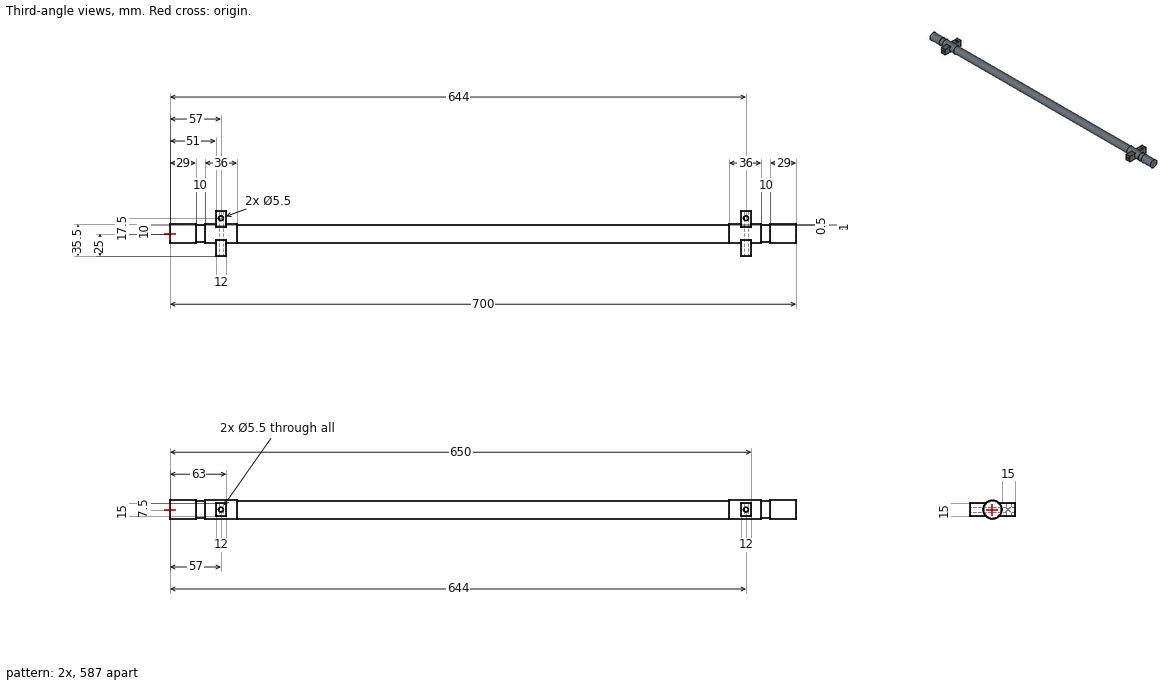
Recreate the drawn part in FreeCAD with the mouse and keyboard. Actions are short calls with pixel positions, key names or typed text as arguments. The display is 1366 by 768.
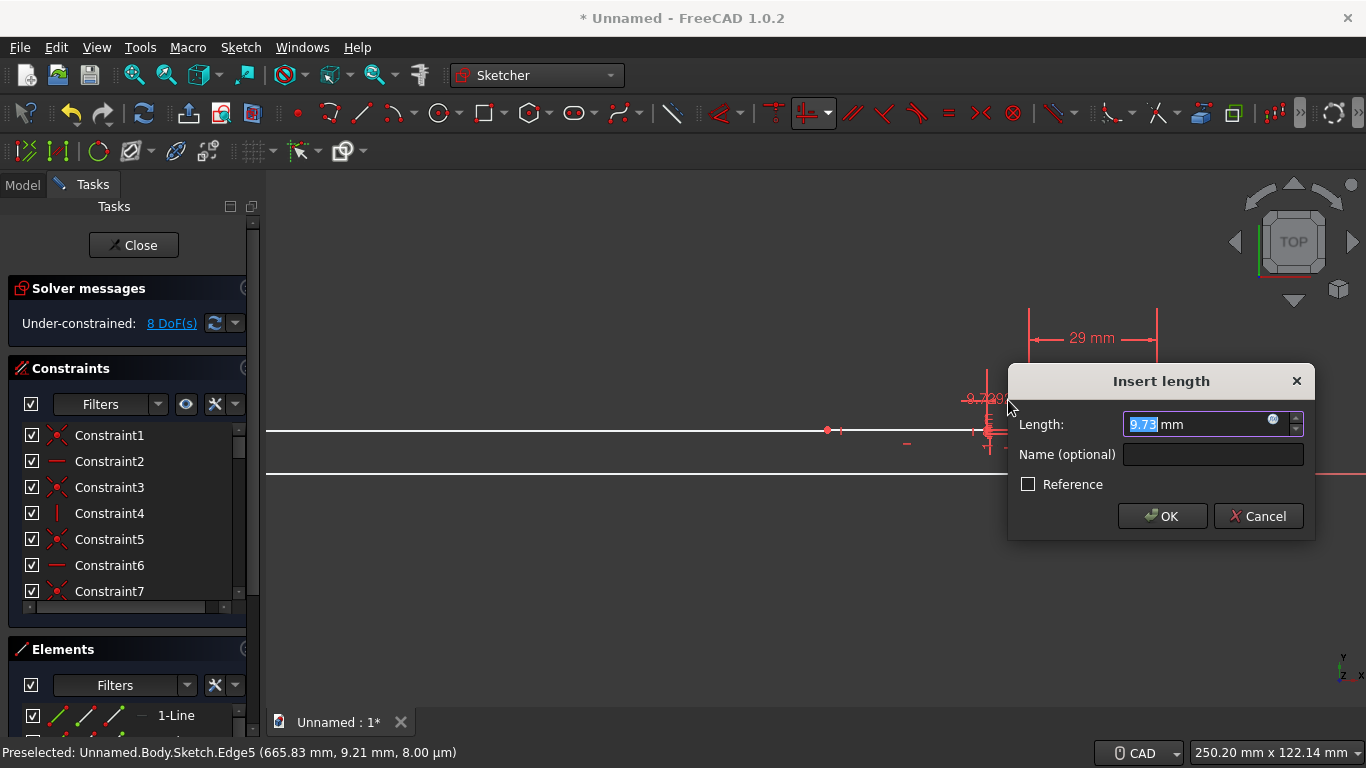
text(10)
key(Return)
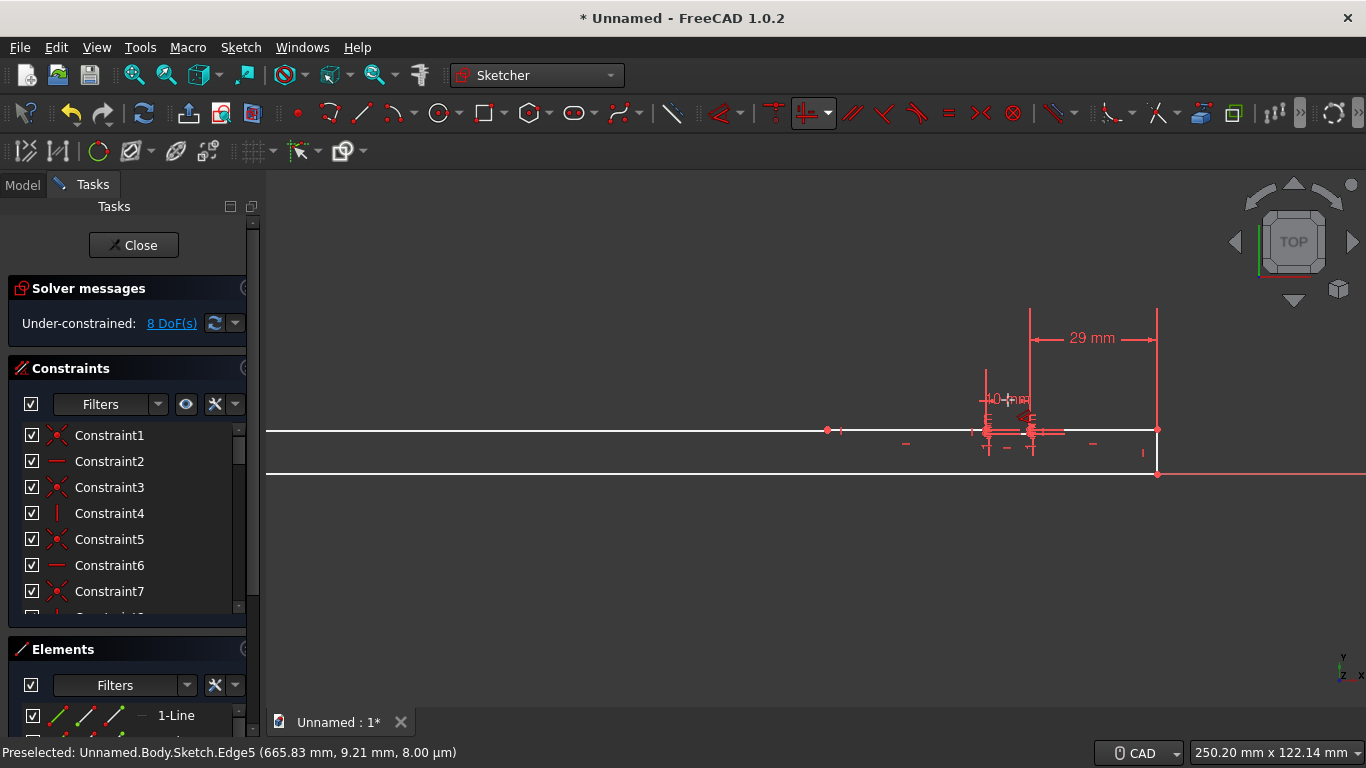
scroll(1033, 435, down, 8)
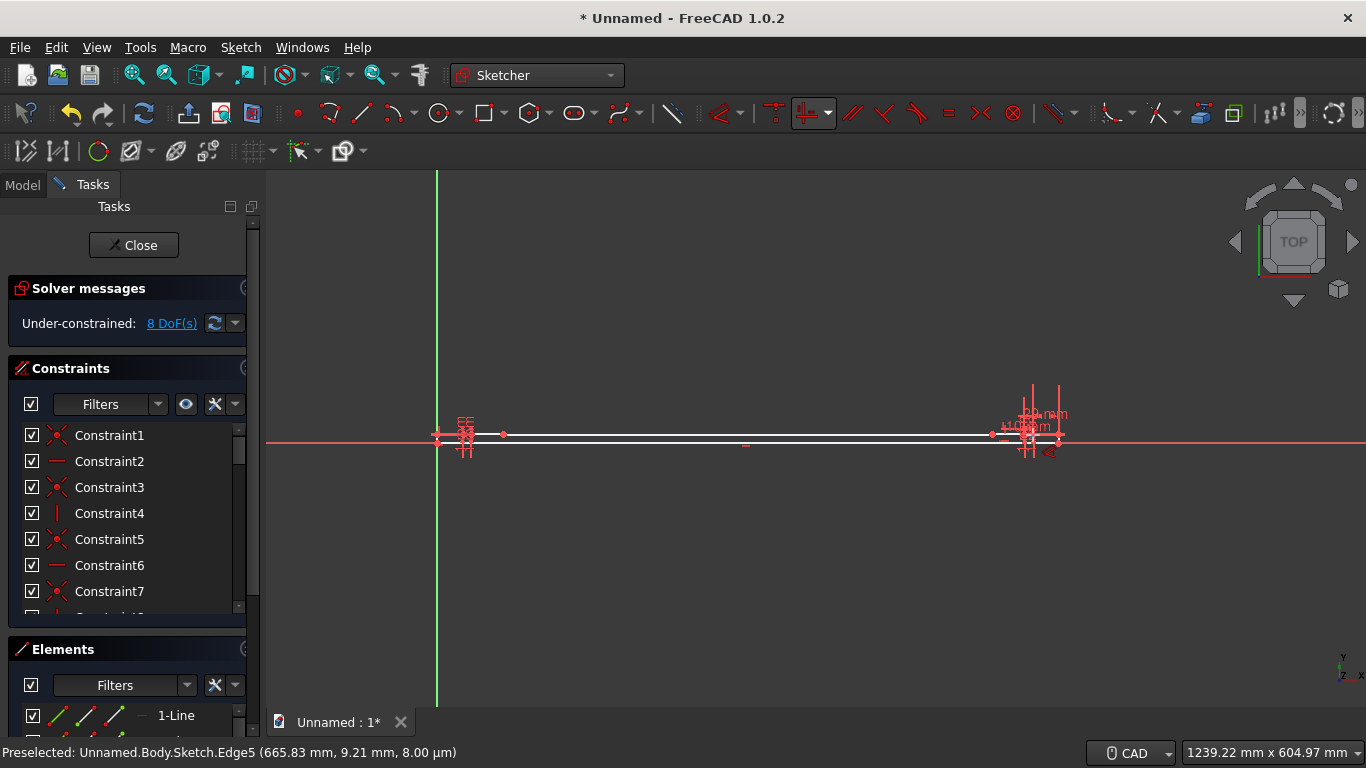
scroll(1014, 434, up, 3)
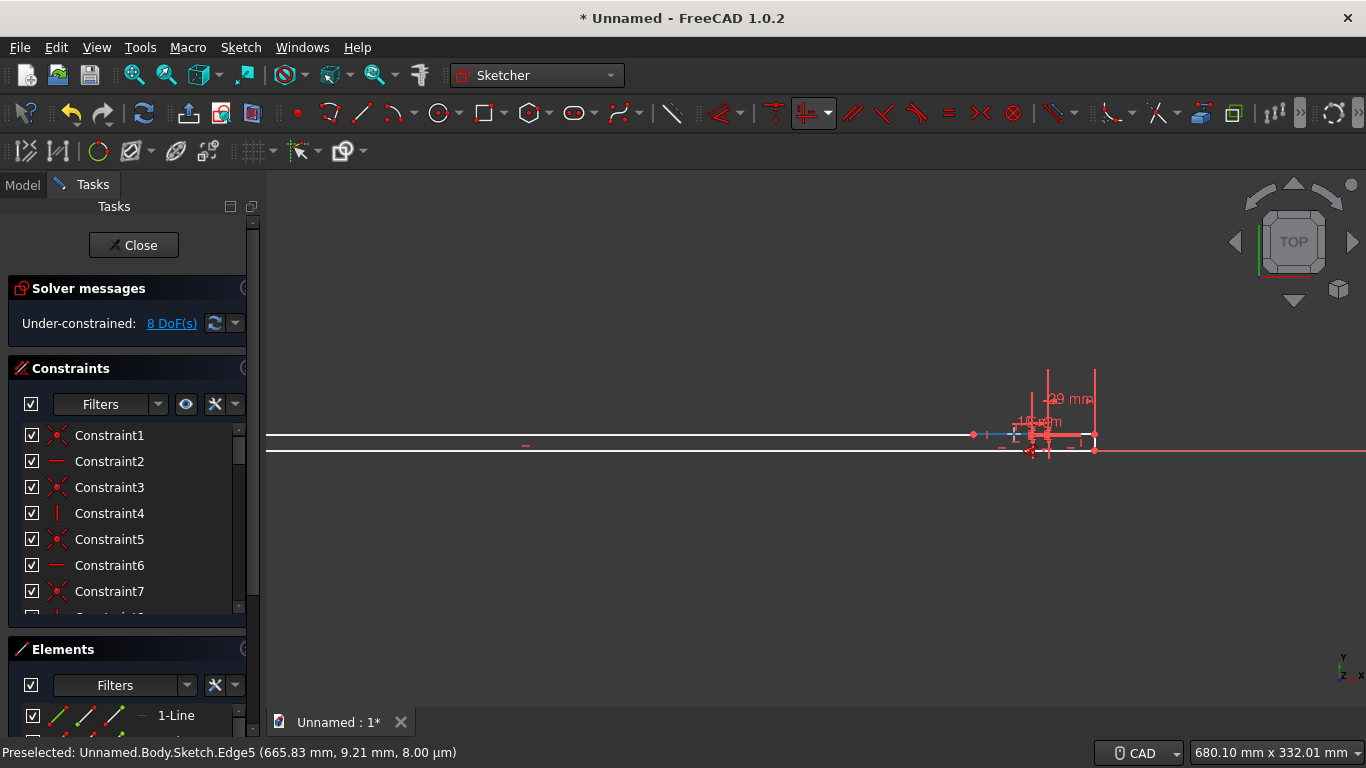
click(1014, 434)
click(989, 400)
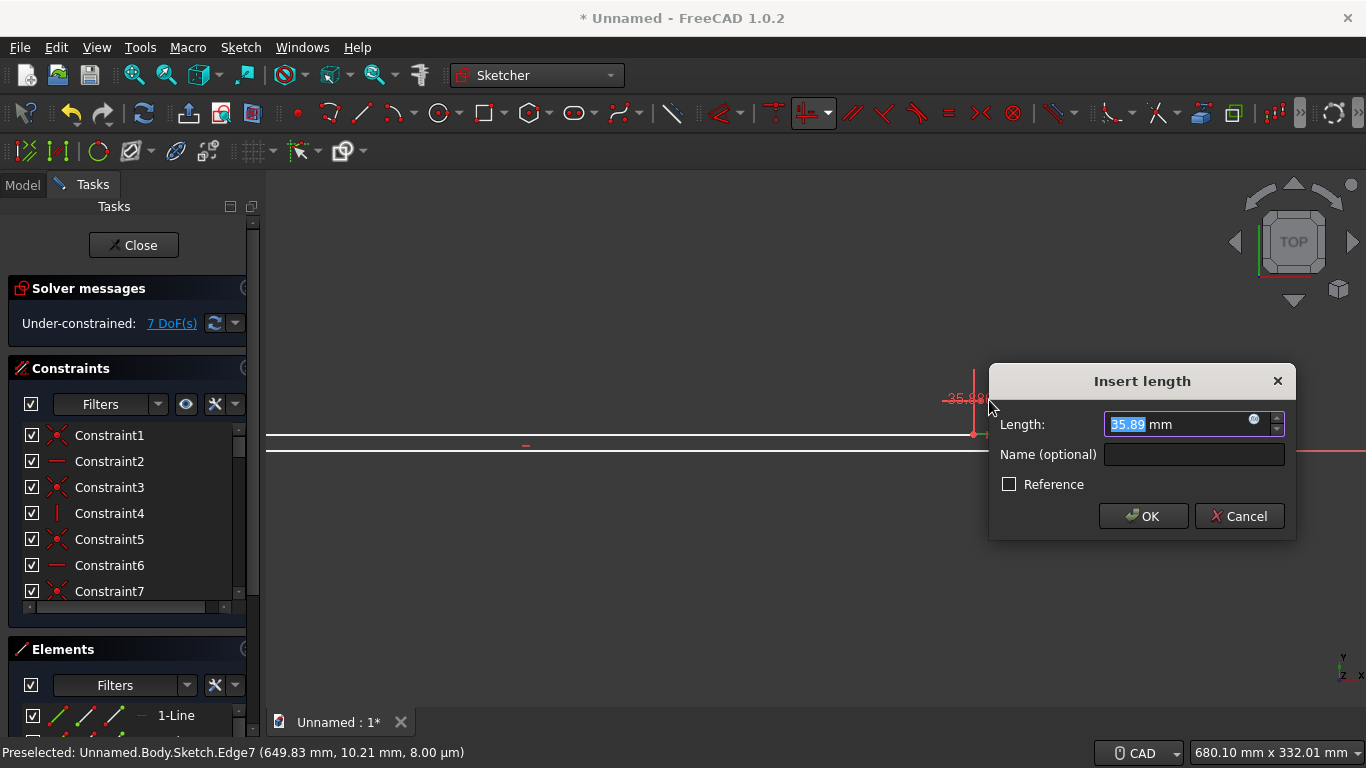
text(36)
key(Return)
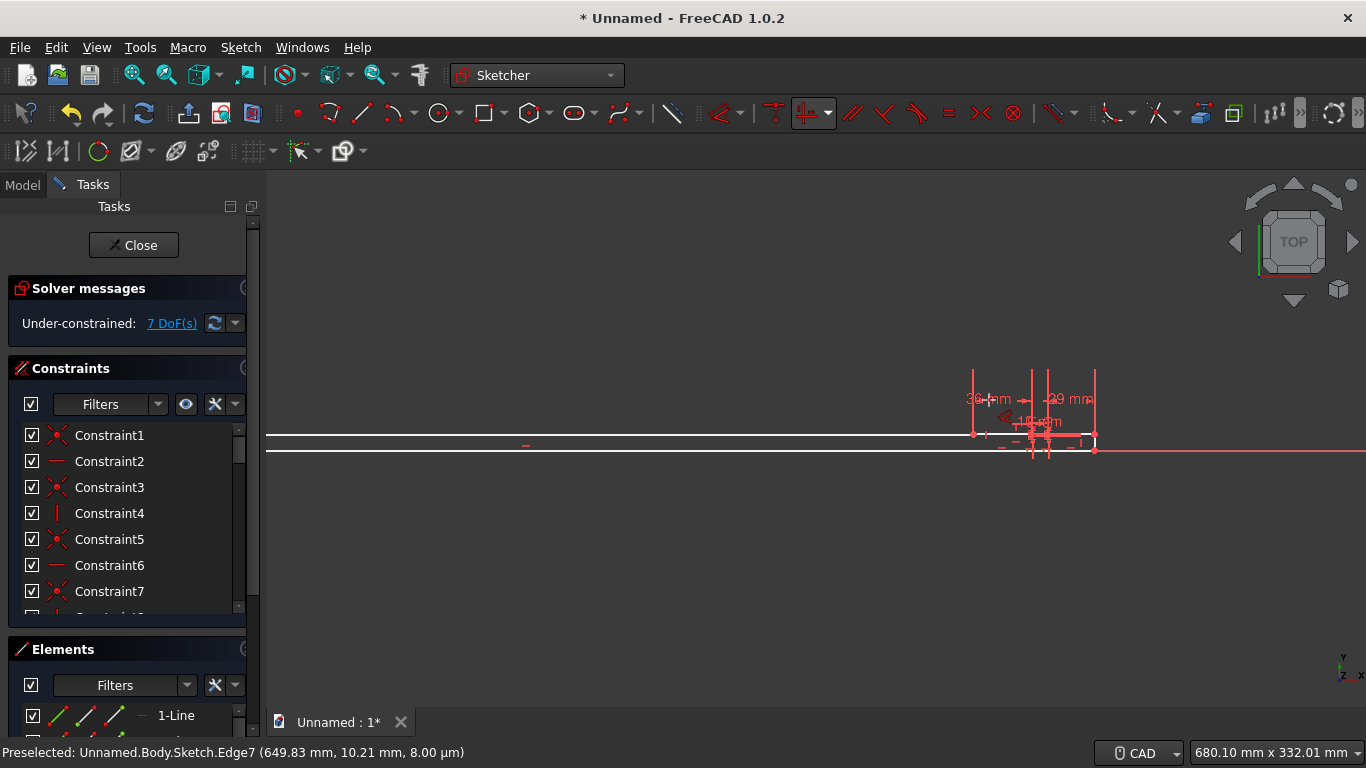
scroll(1013, 434, down, 3)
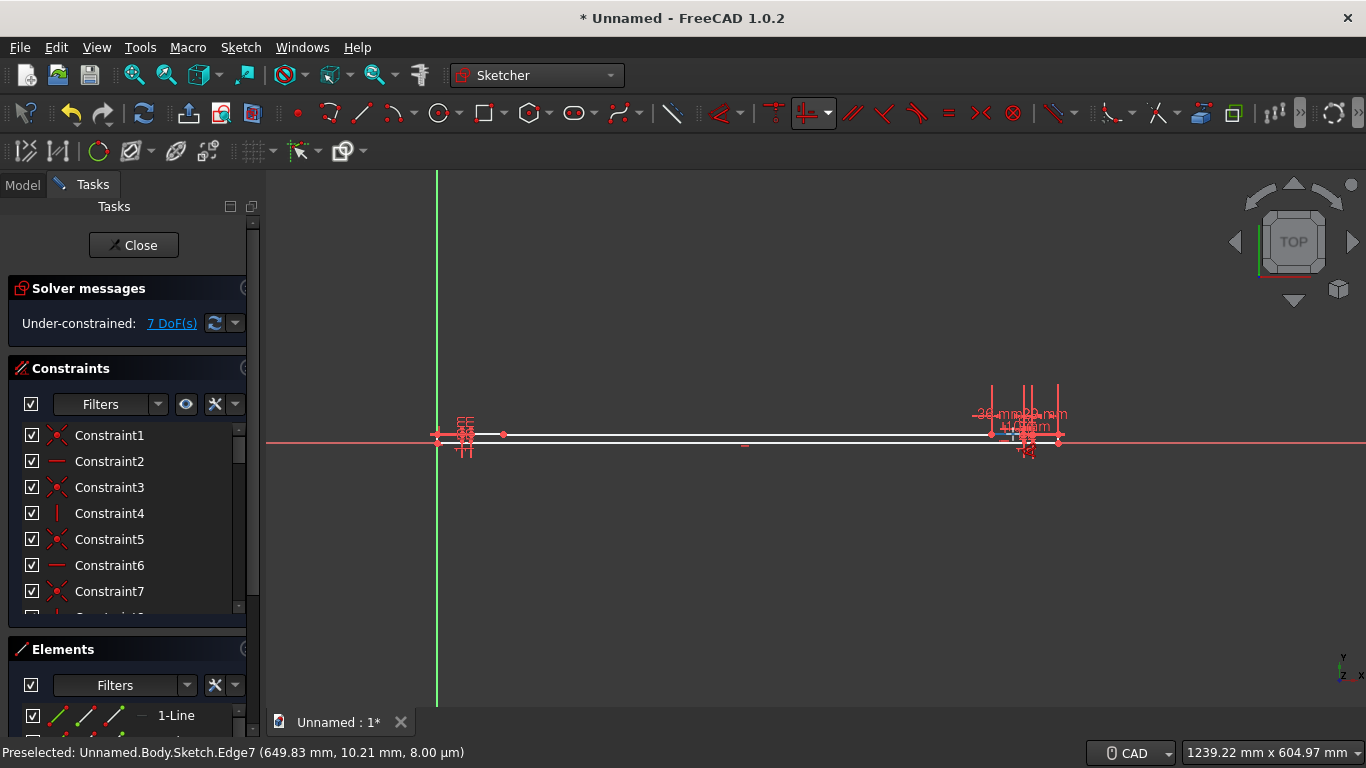
scroll(494, 434, up, 2)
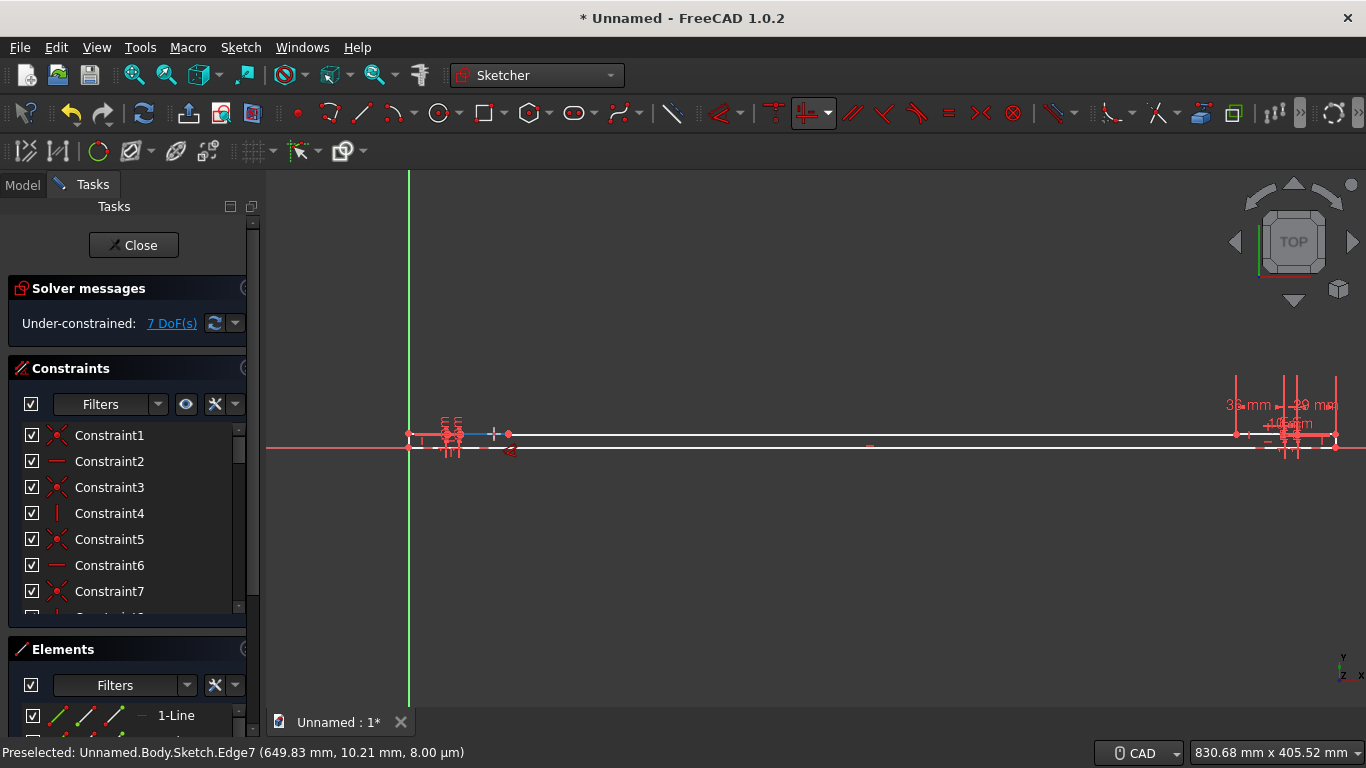
click(494, 434)
click(484, 400)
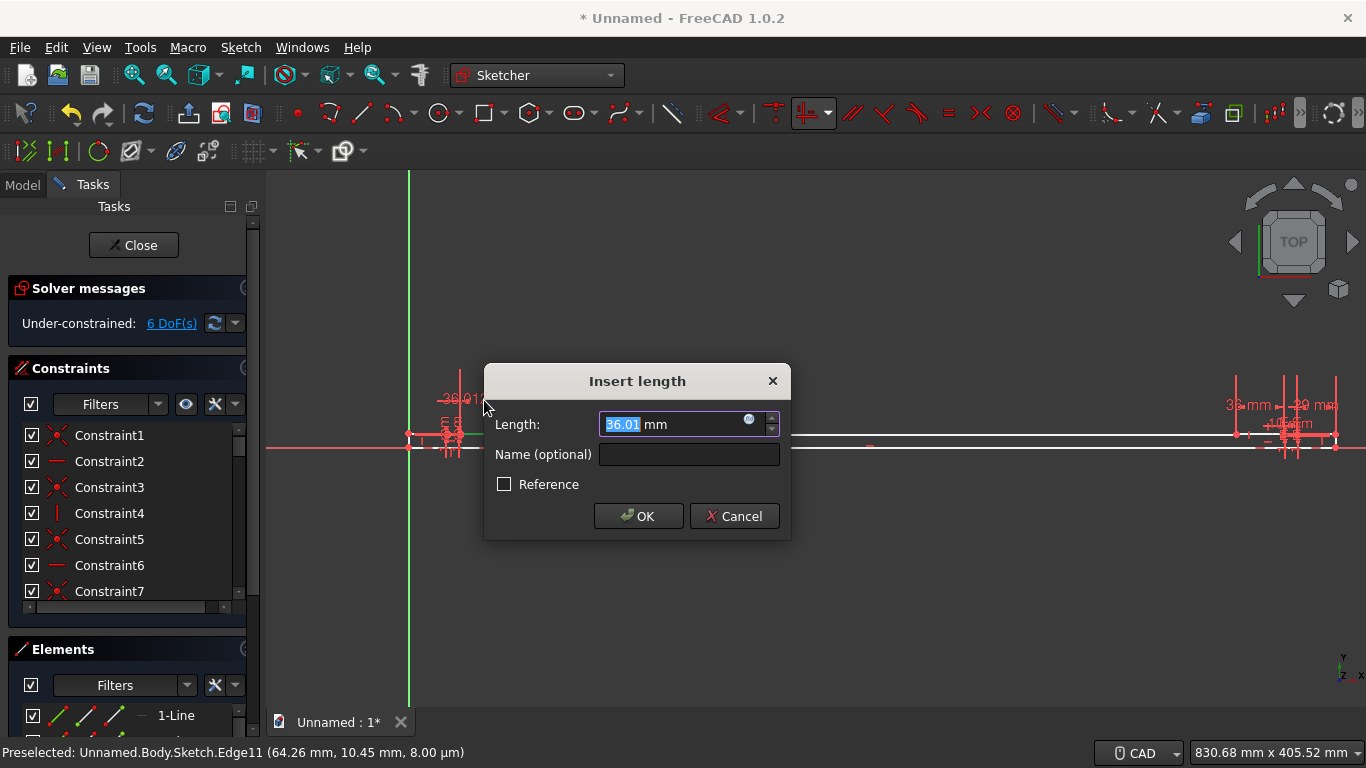
text(36)
key(Return)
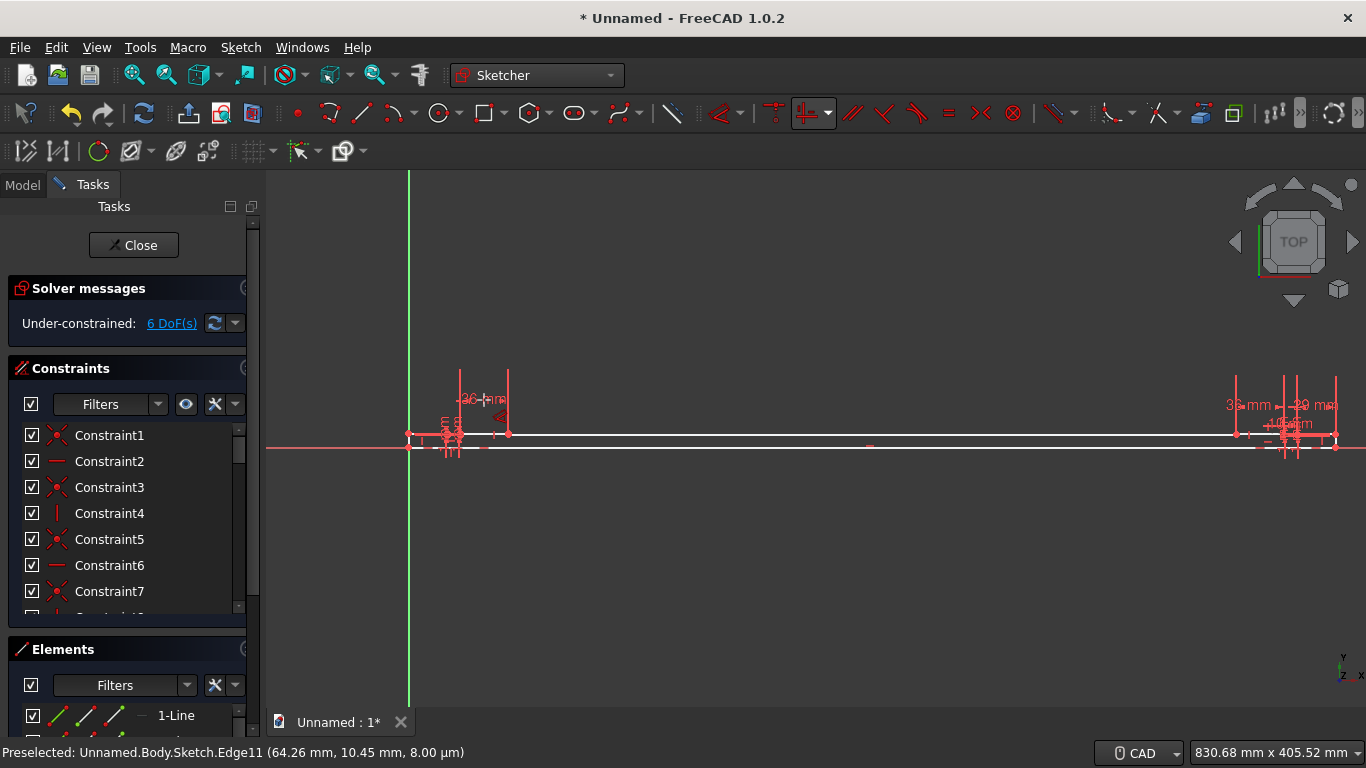
scroll(454, 435, up, 6)